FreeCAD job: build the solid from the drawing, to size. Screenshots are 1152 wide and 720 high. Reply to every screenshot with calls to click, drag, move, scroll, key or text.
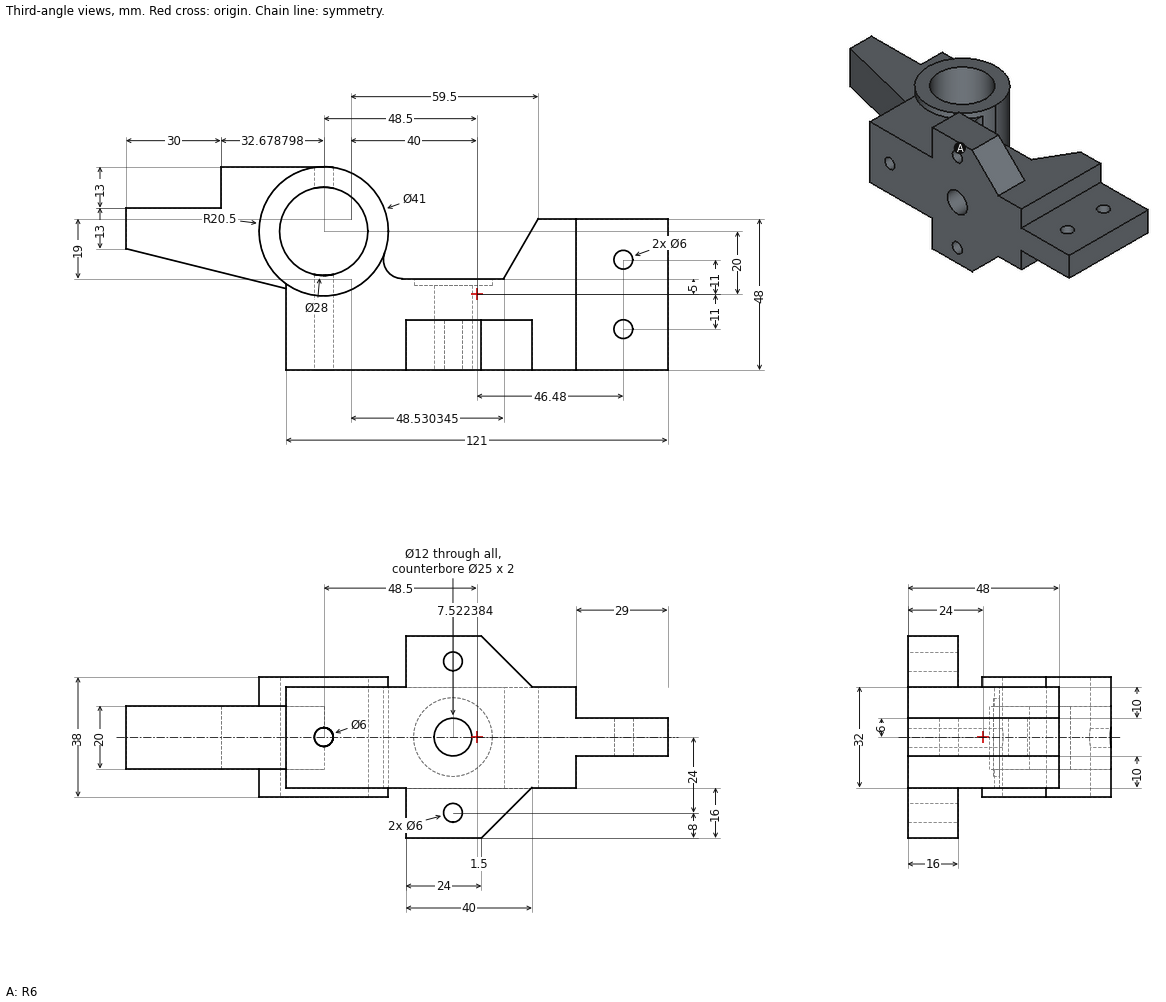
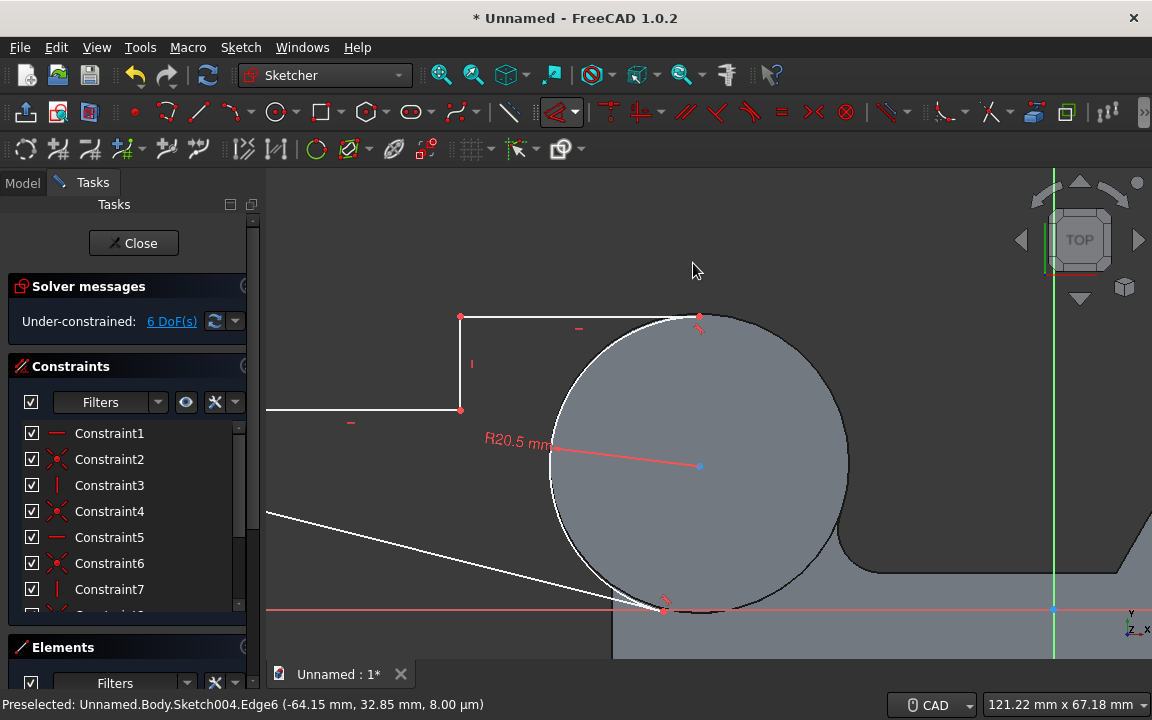
click(460, 345)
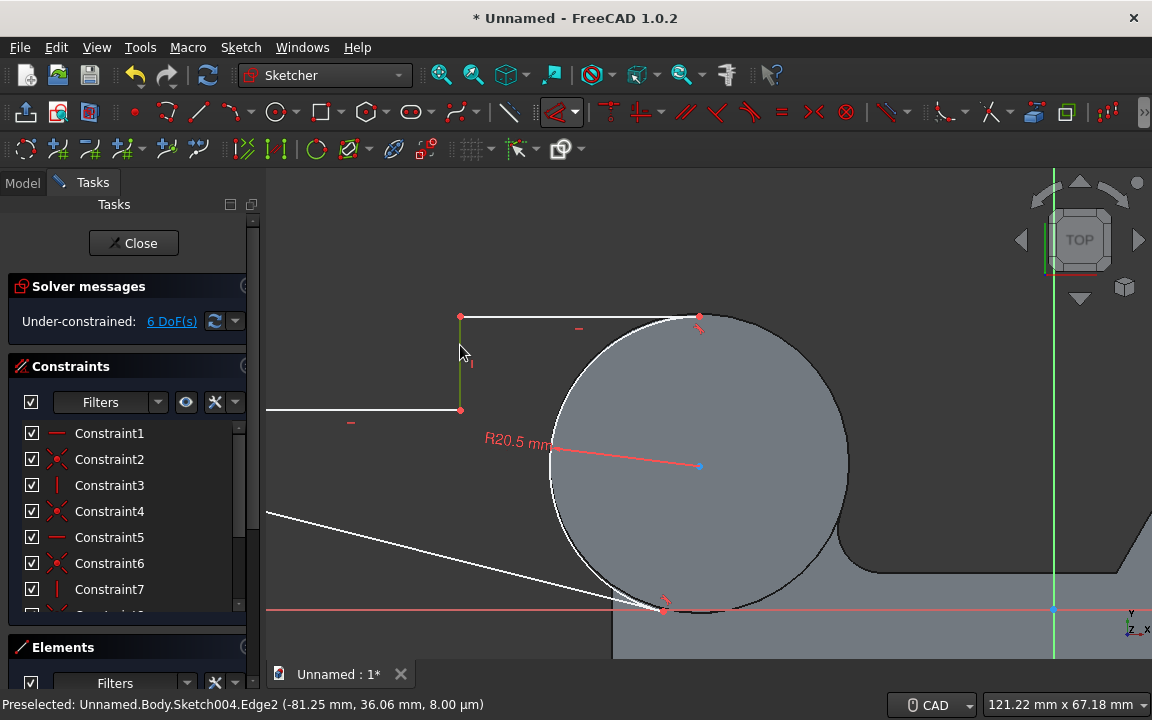
key(i)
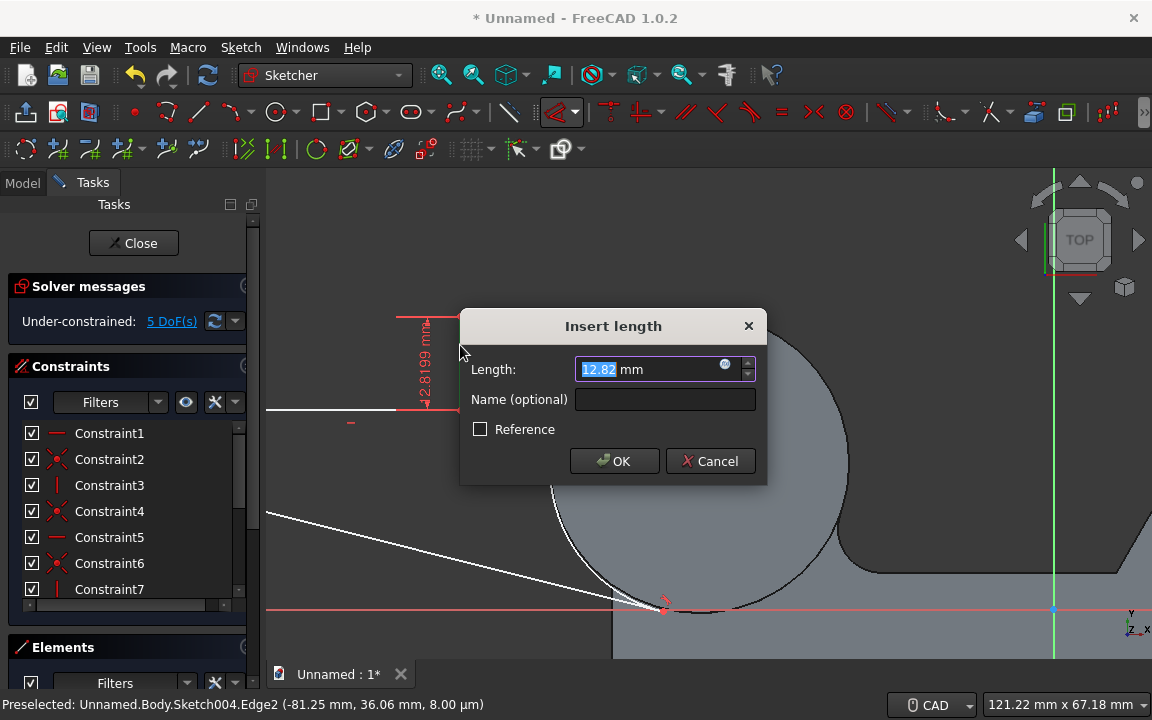
text(13)
key(Return)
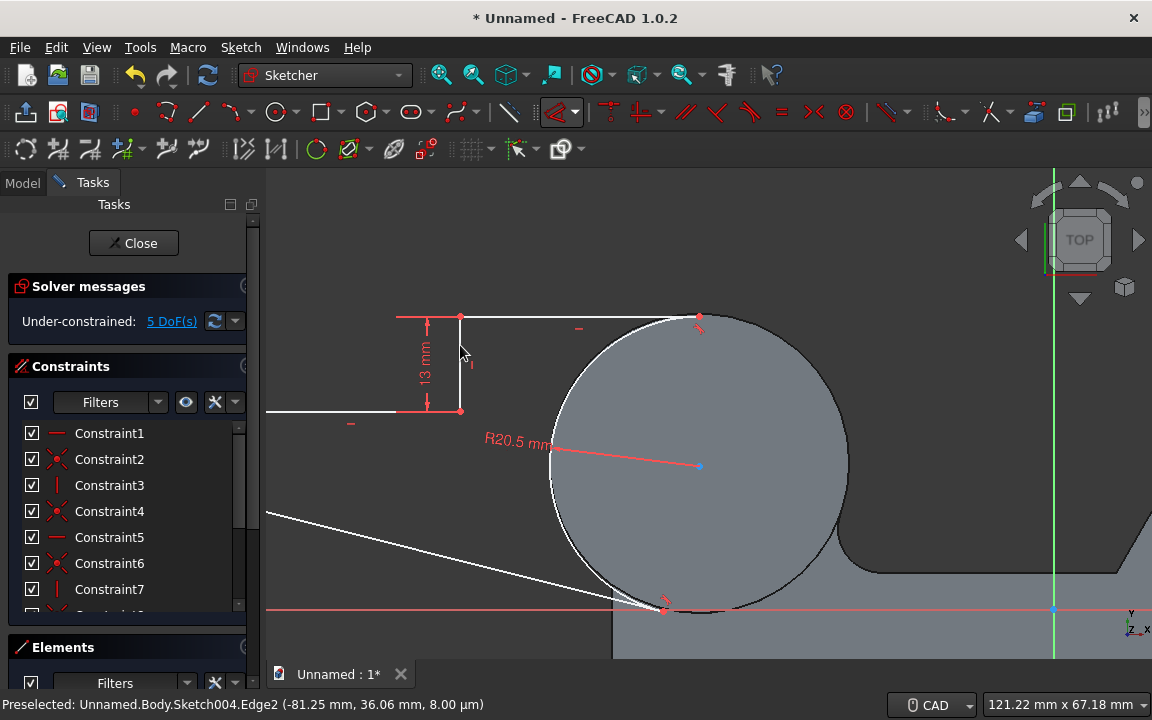
click(395, 412)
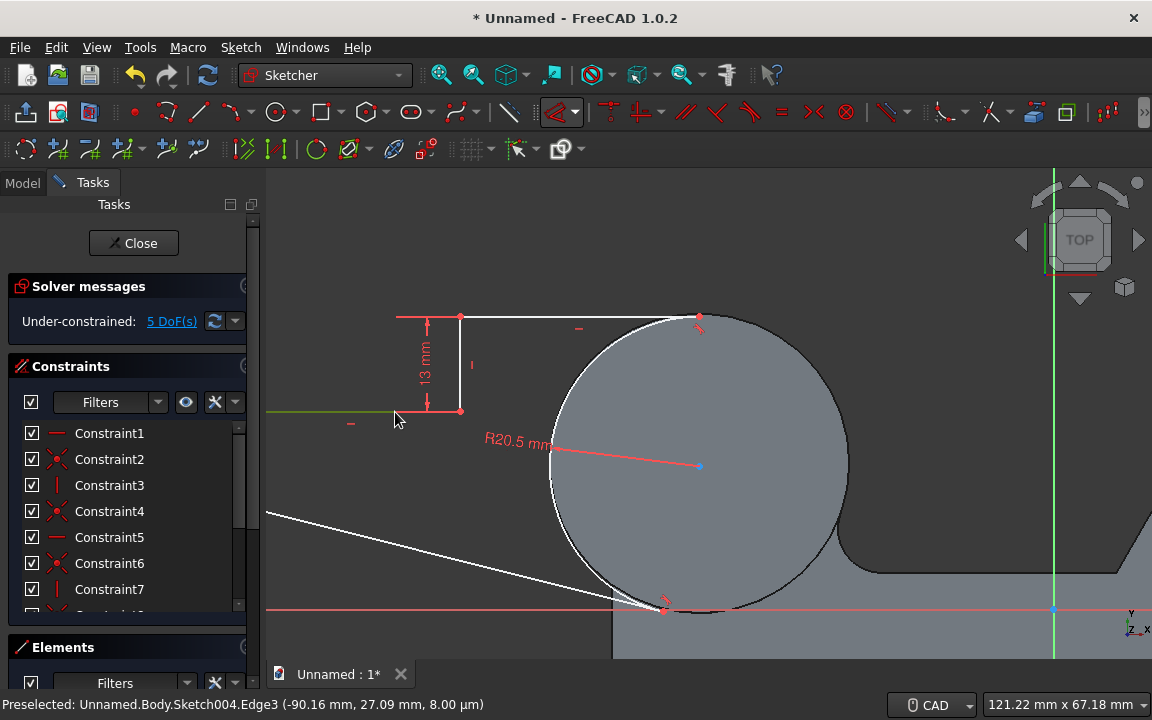
key(l)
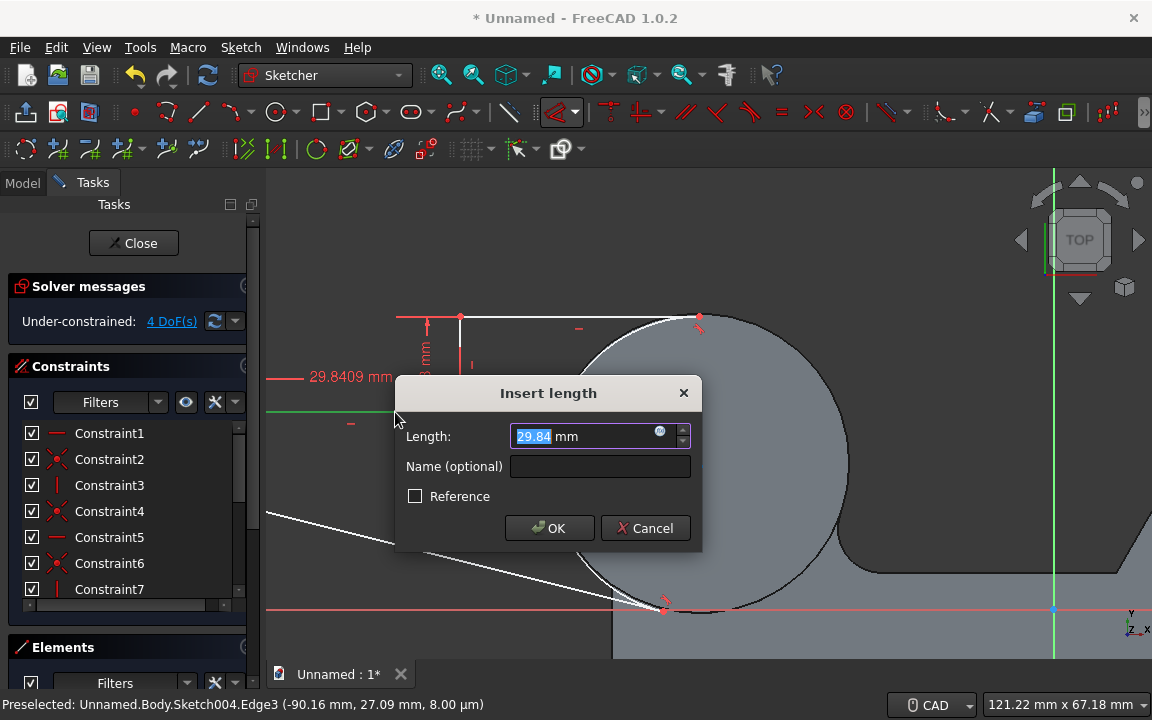
text(30)
key(Return)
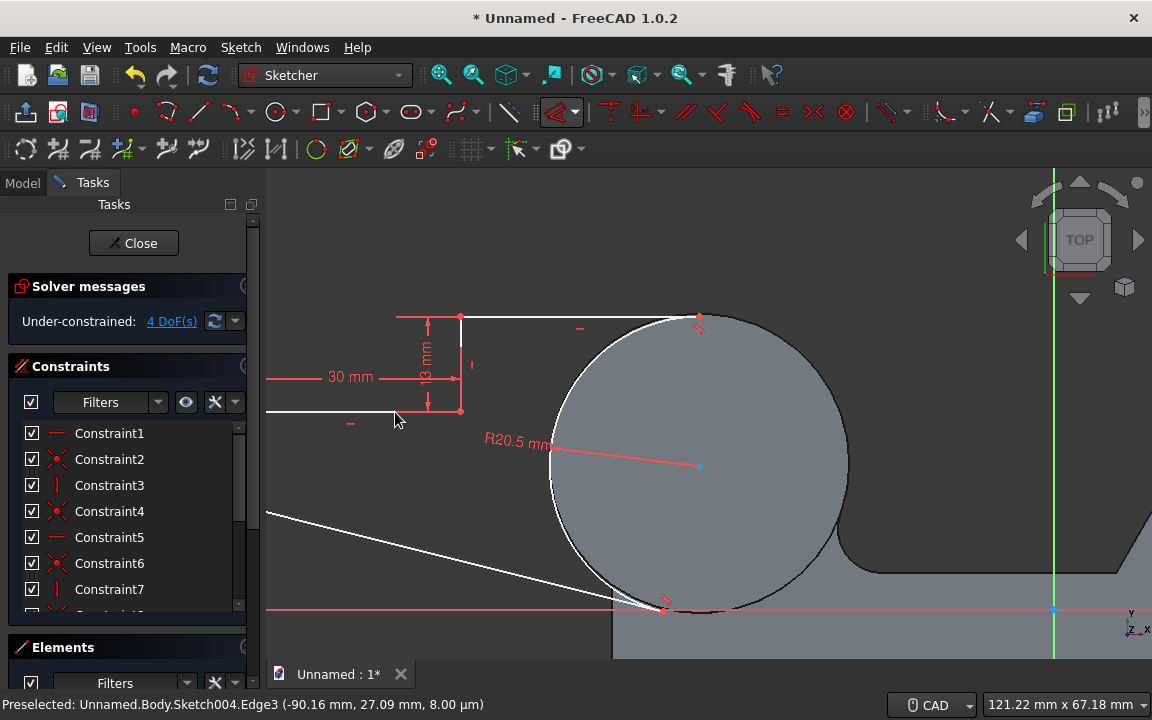
scroll(632, 355, down, 3)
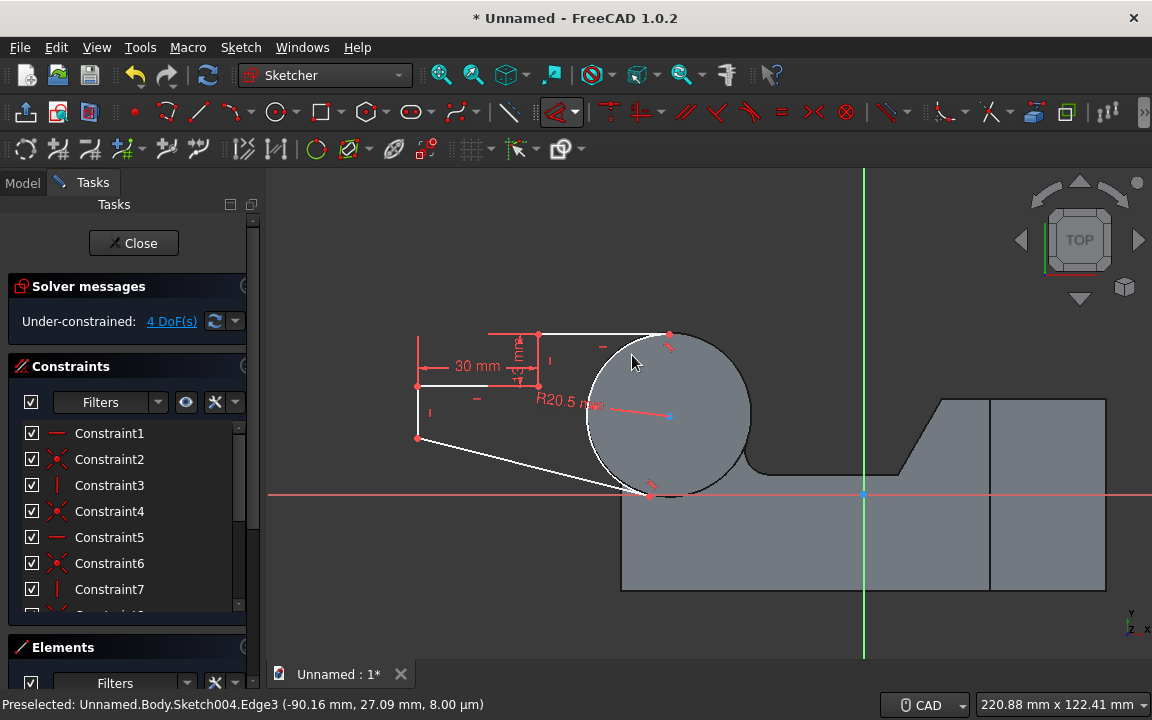
click(418, 402)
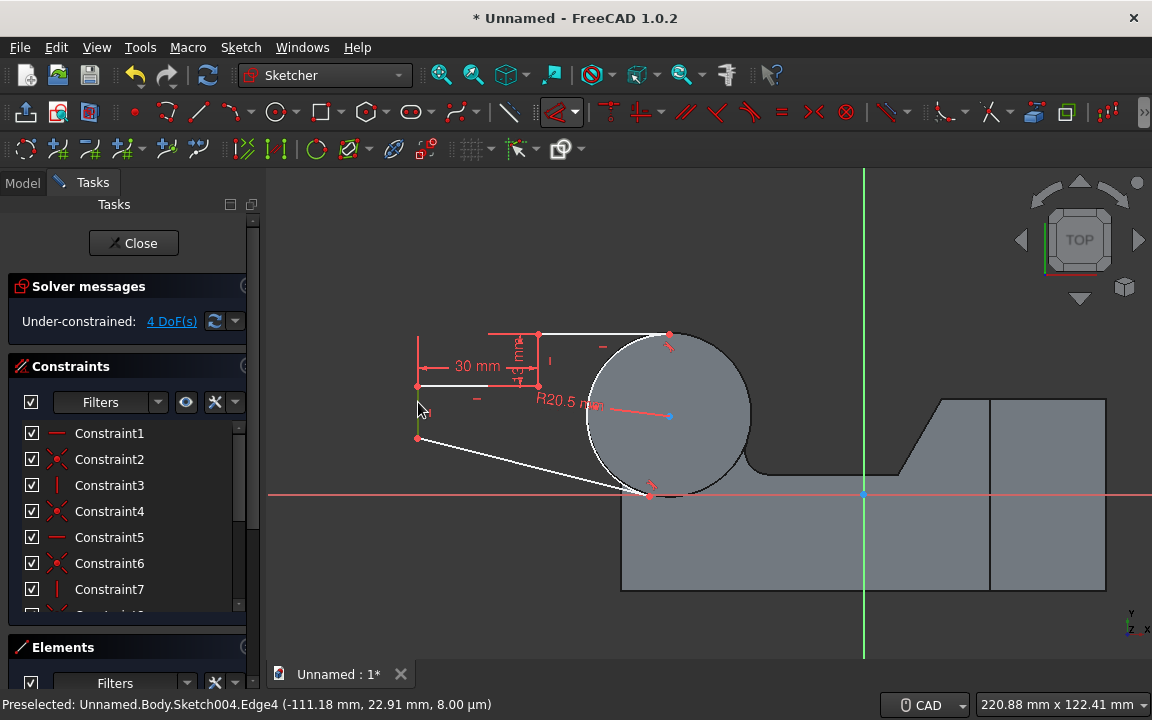
key(i)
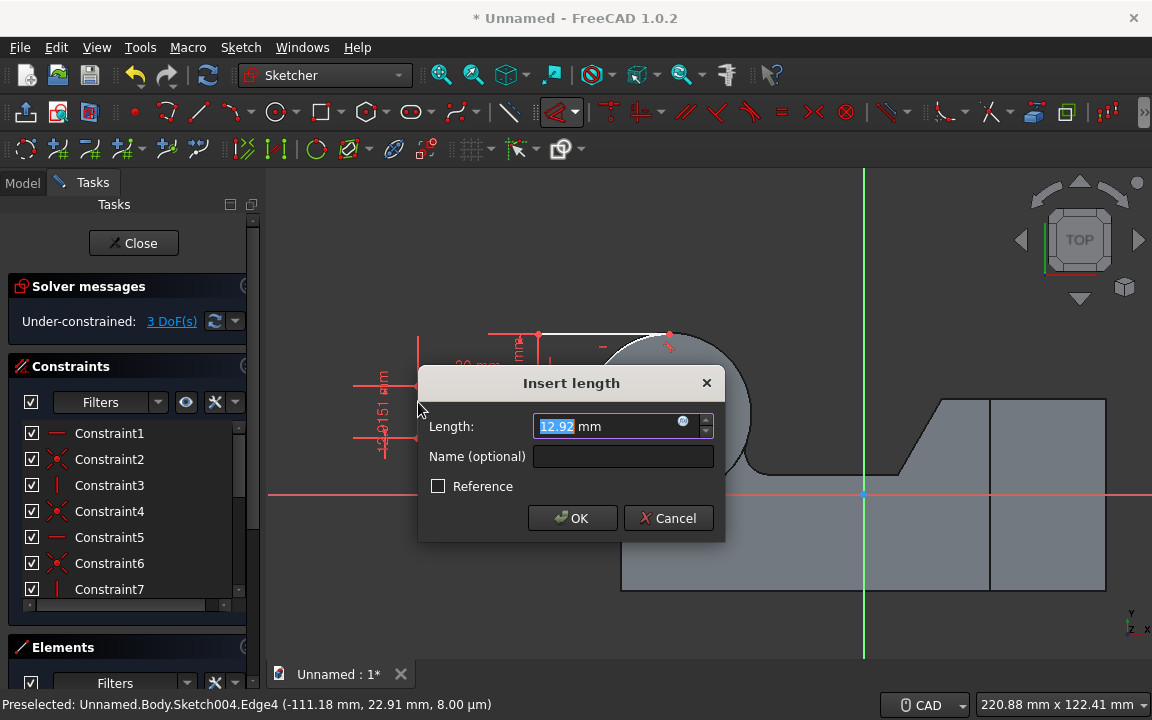
text(13)
key(Return)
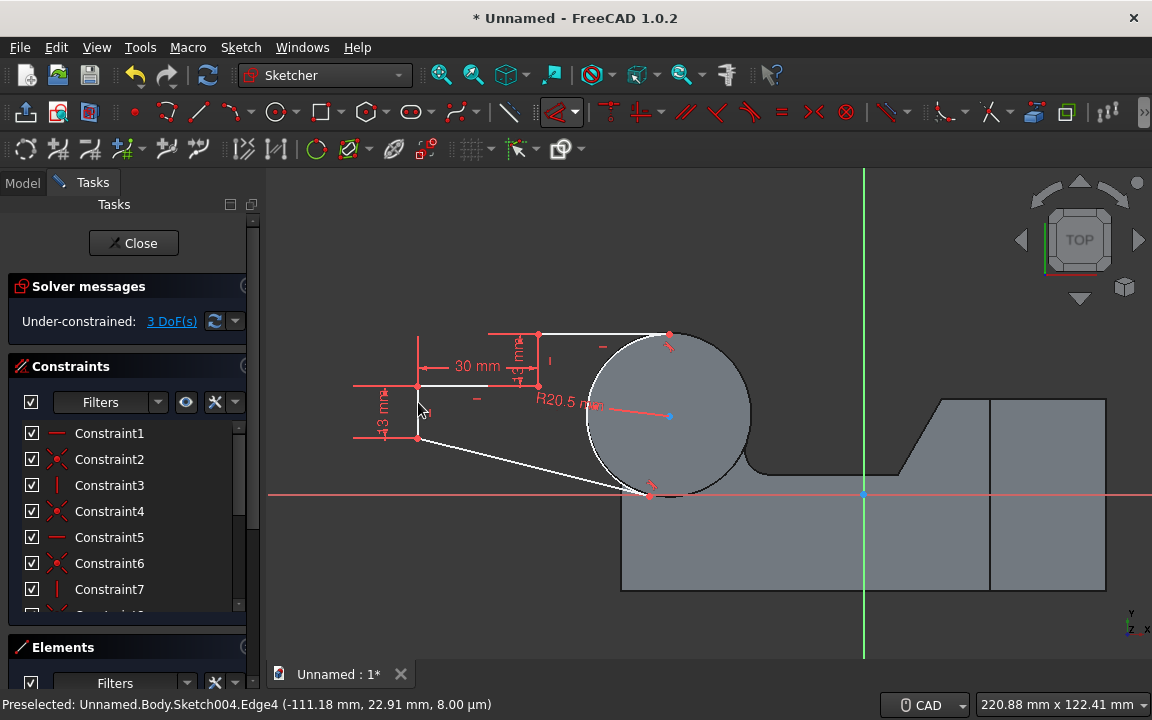
click(669, 416)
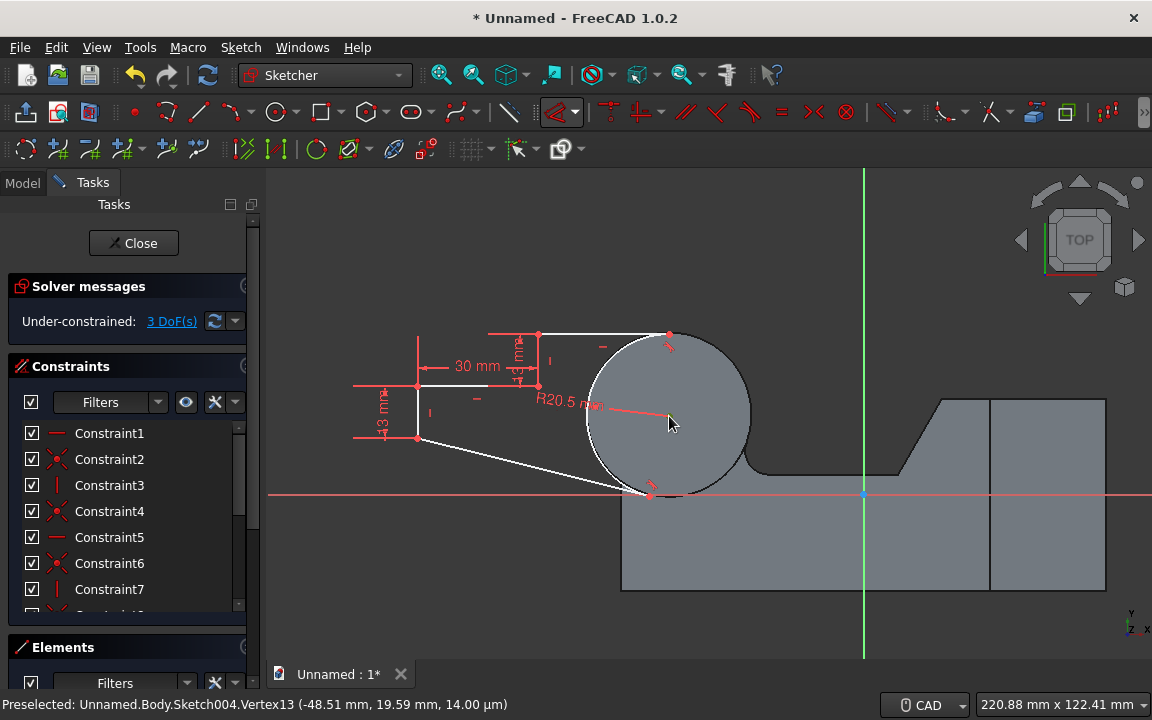
click(578, 112)